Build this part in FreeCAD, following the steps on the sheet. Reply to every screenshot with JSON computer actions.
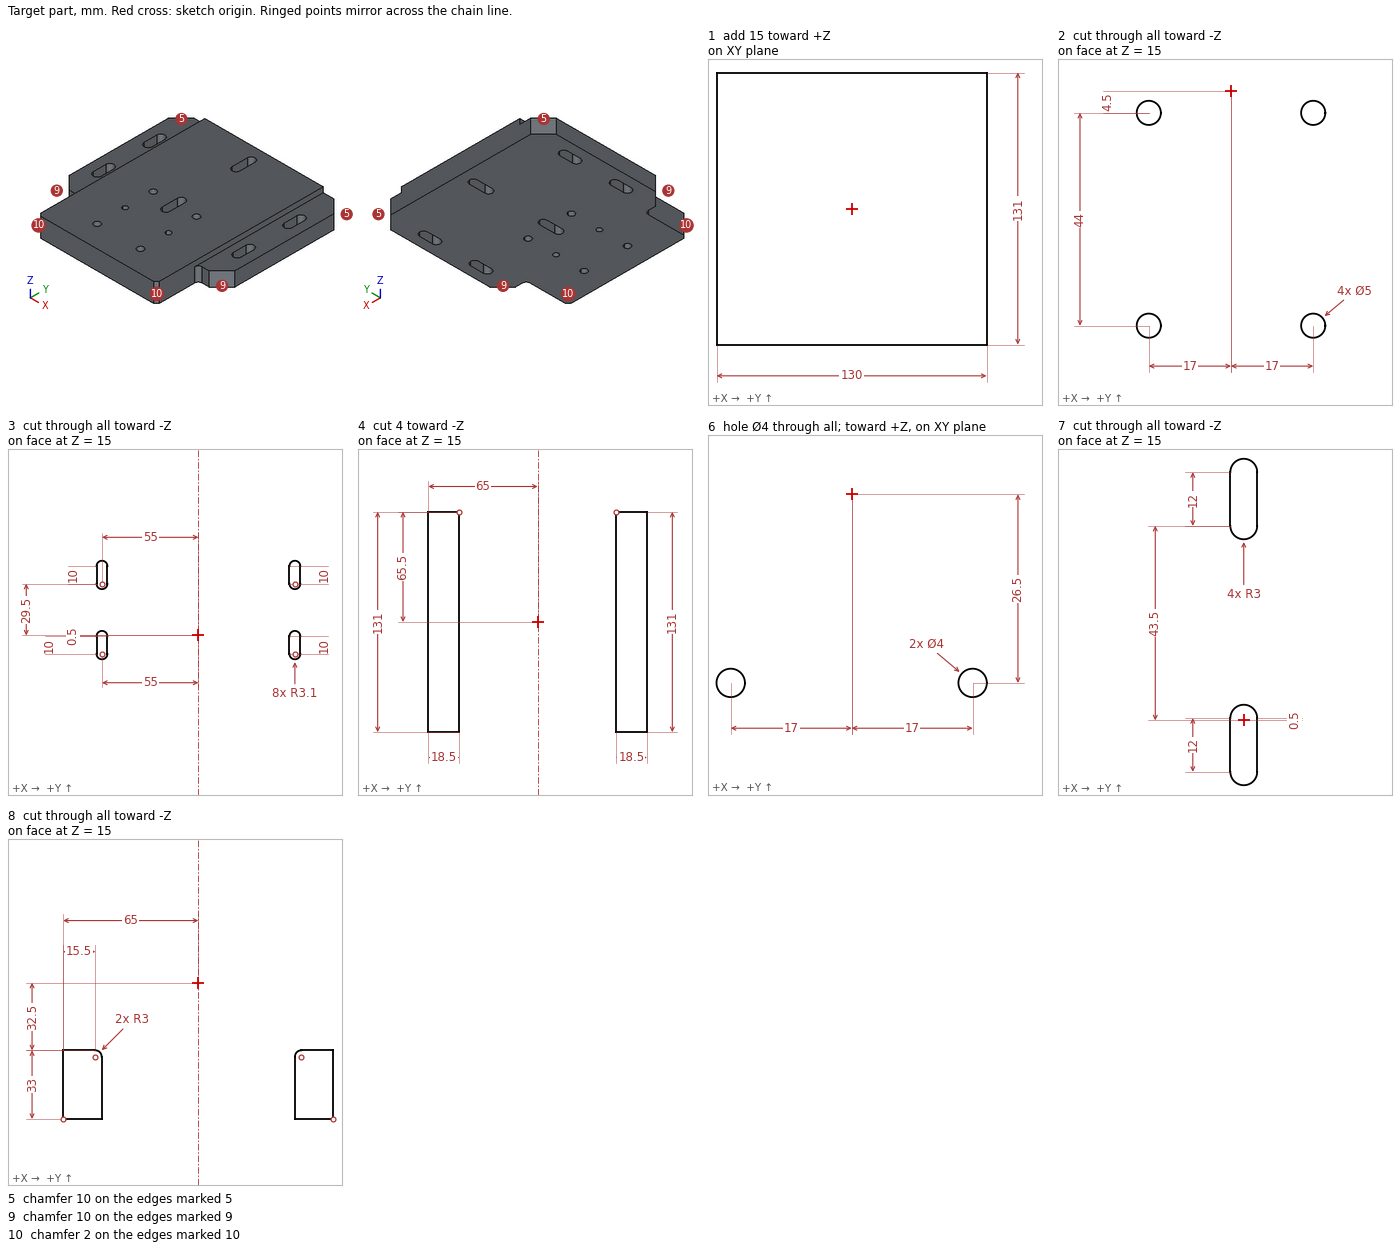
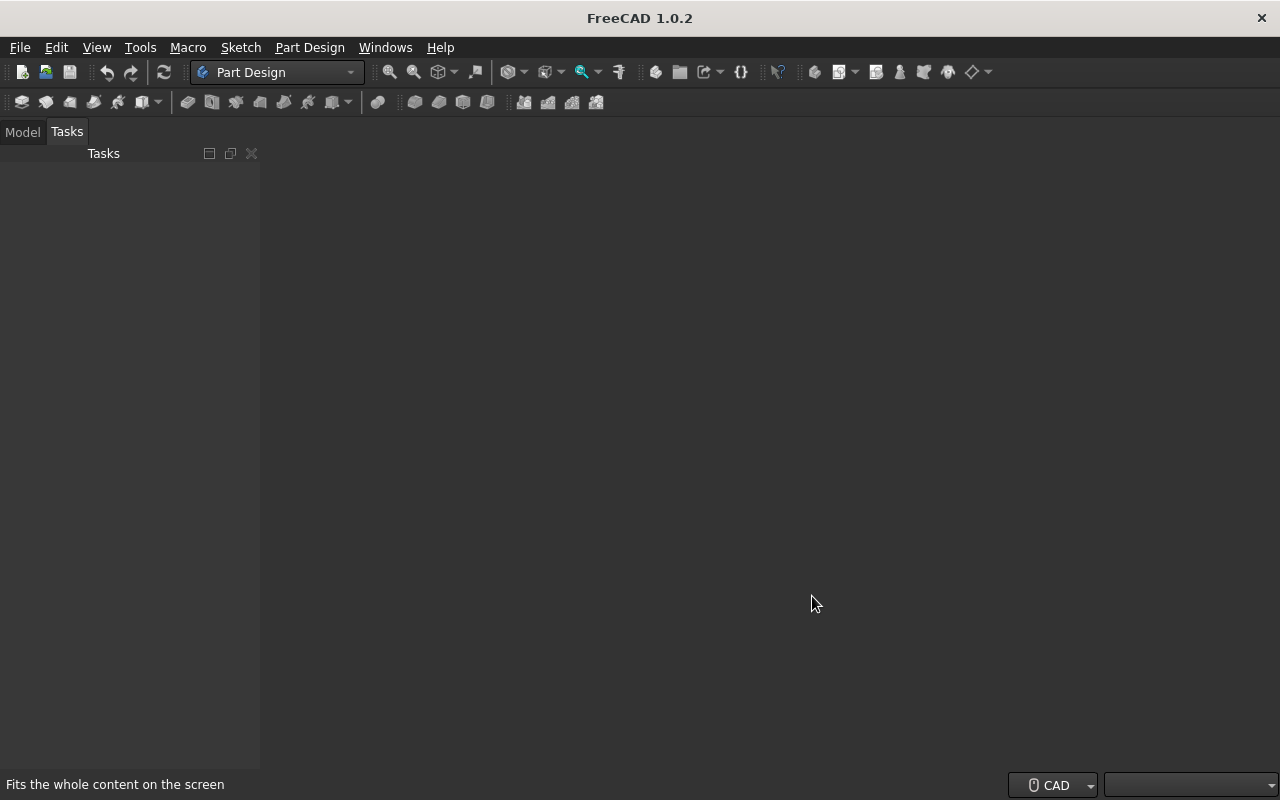
{"action": "key", "text": "ctrl+n"}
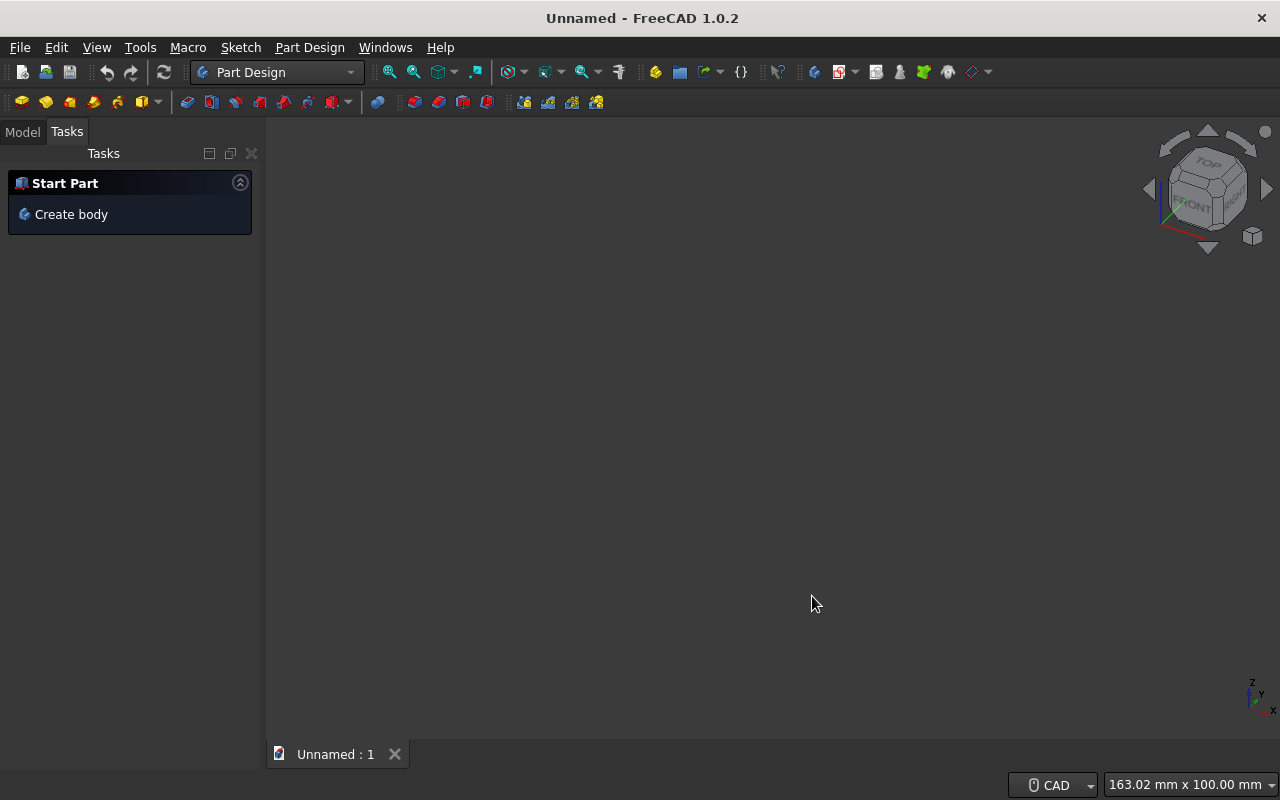
{"action": "left_click", "coordinate": [840, 72]}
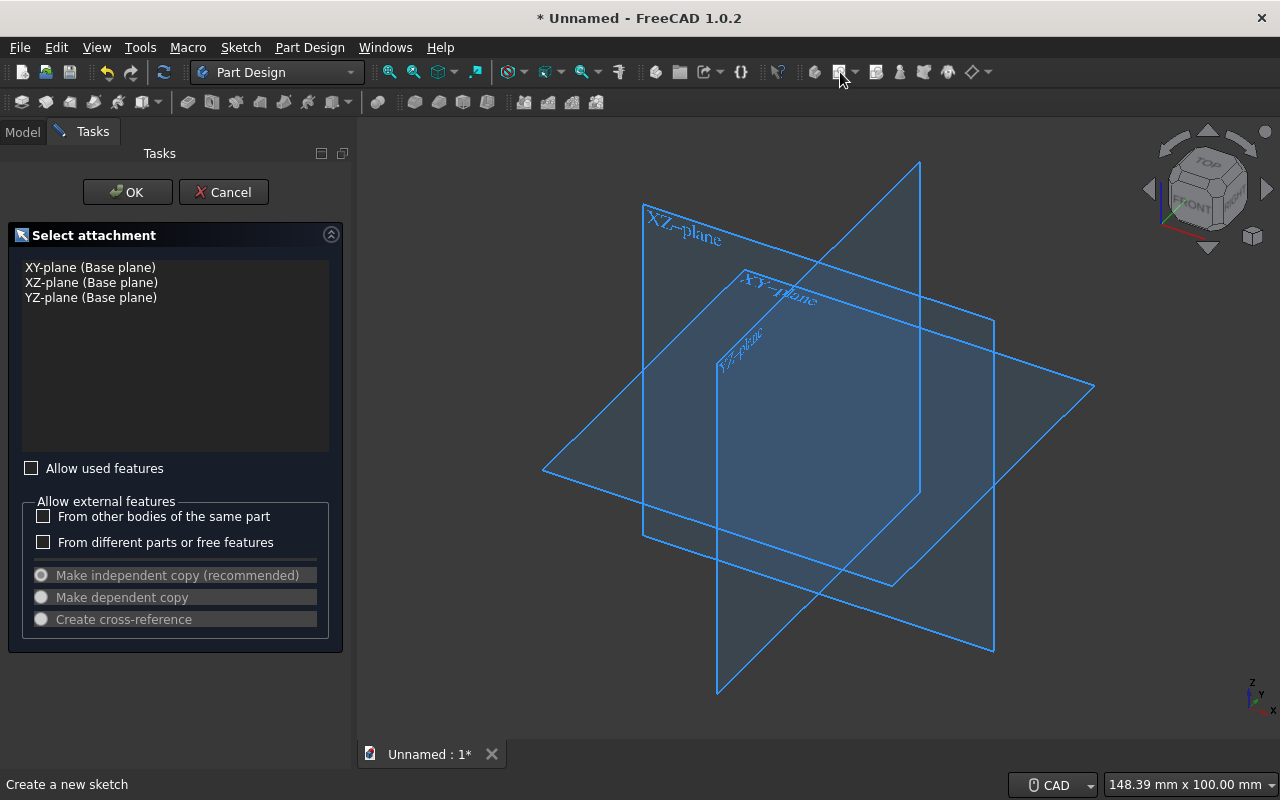
{"action": "left_click", "coordinate": [82, 268]}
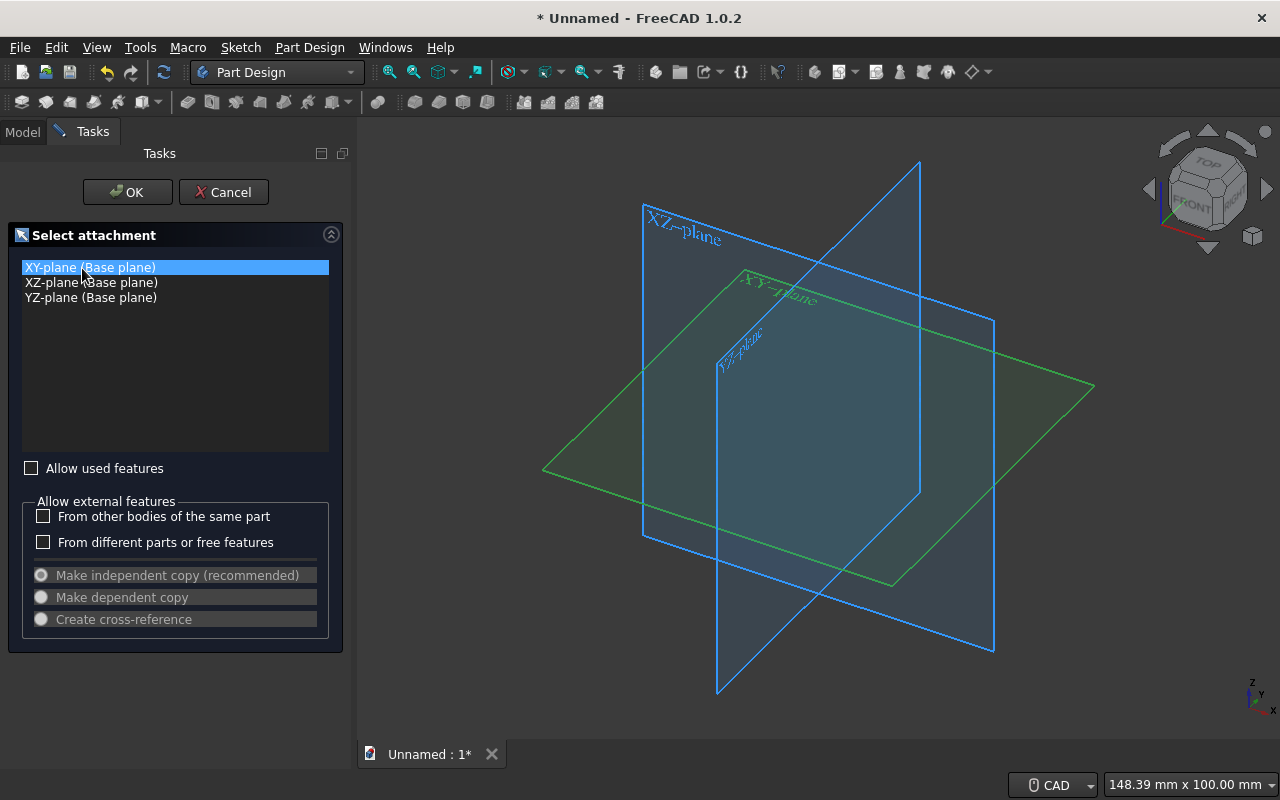
{"action": "left_click", "coordinate": [128, 192]}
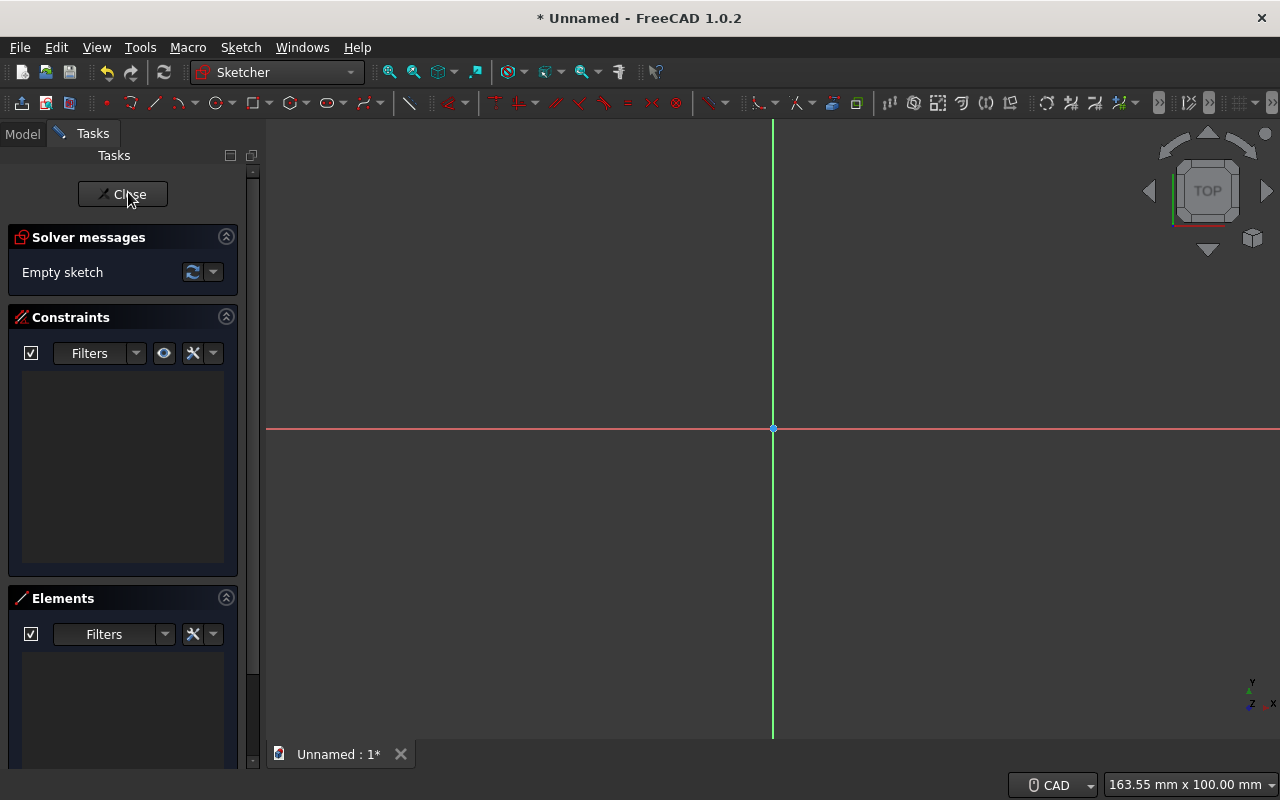
{"action": "scroll", "coordinate": [649, 429], "scroll_direction": "down", "scroll_amount": 4}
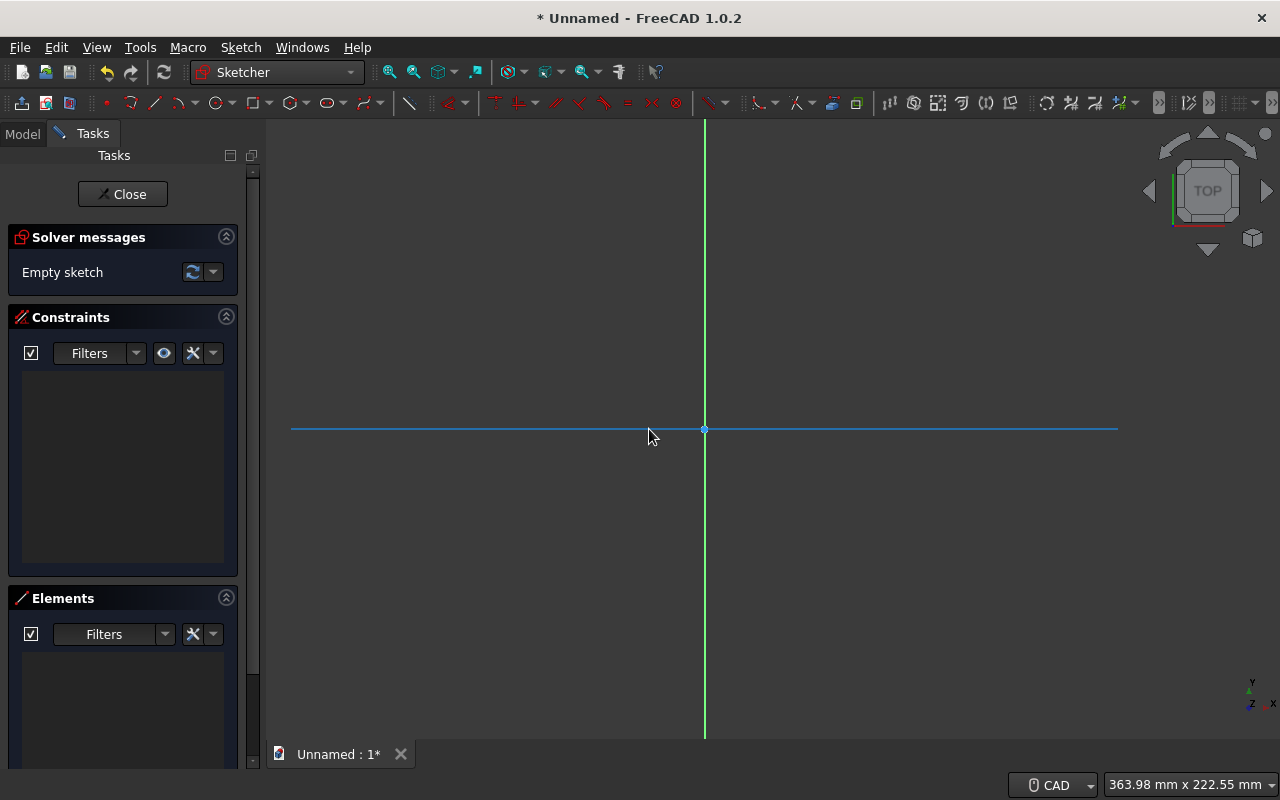
{"action": "left_click", "coordinate": [272, 104]}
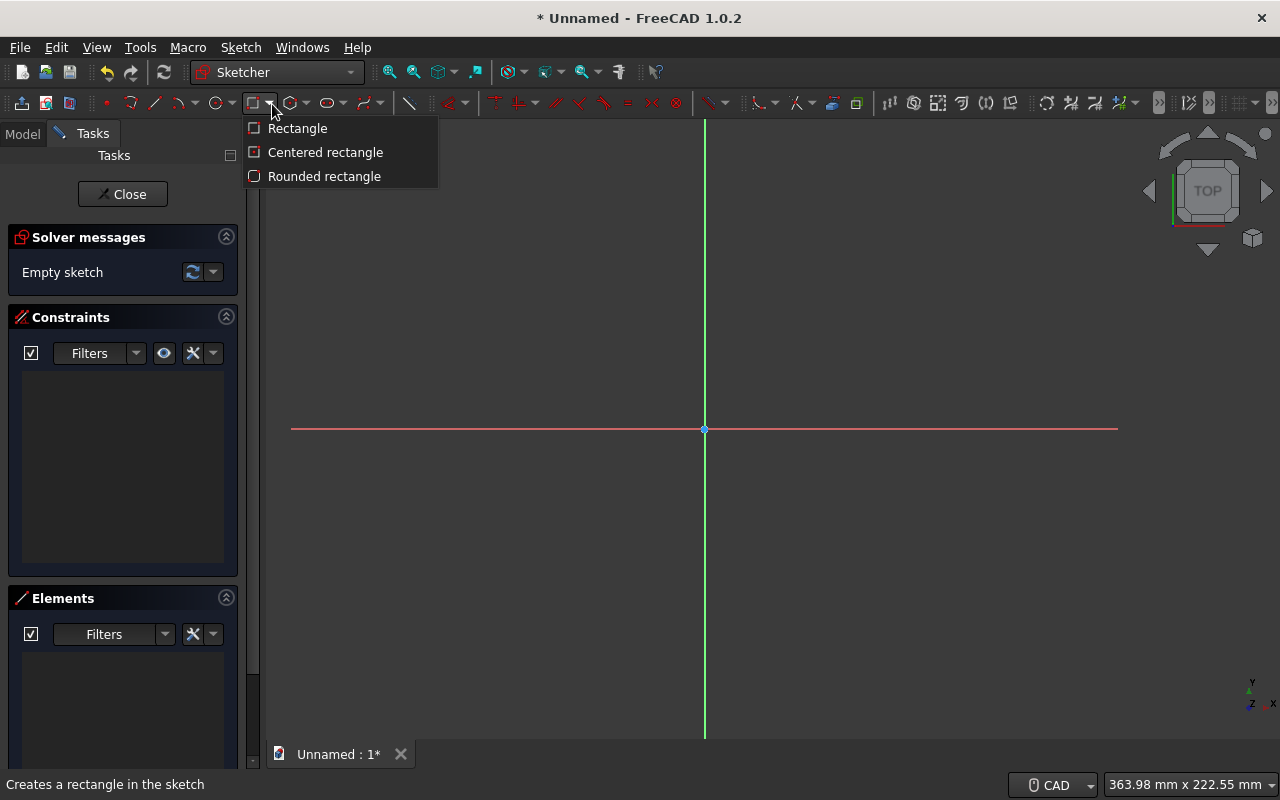
{"action": "left_click", "coordinate": [340, 152]}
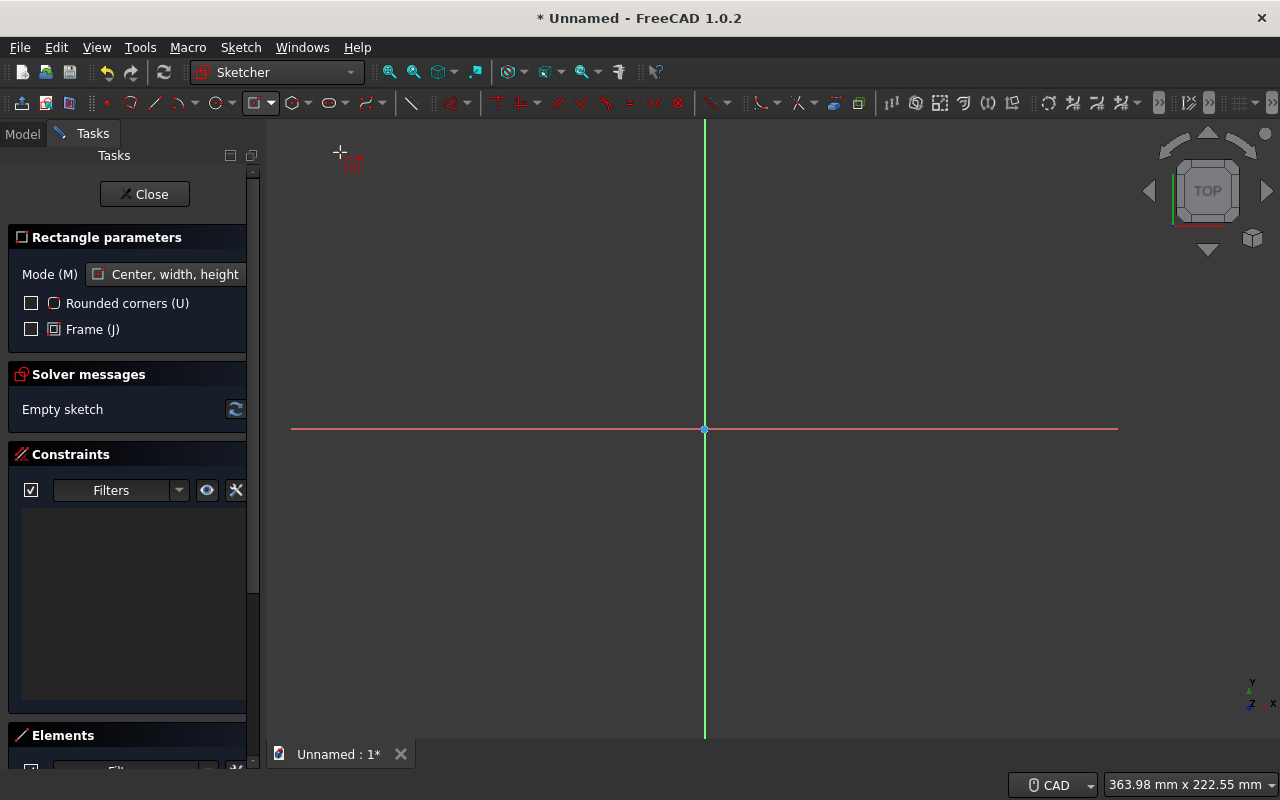
{"action": "left_click", "coordinate": [705, 429]}
{"action": "mouse_move", "coordinate": [886, 247]}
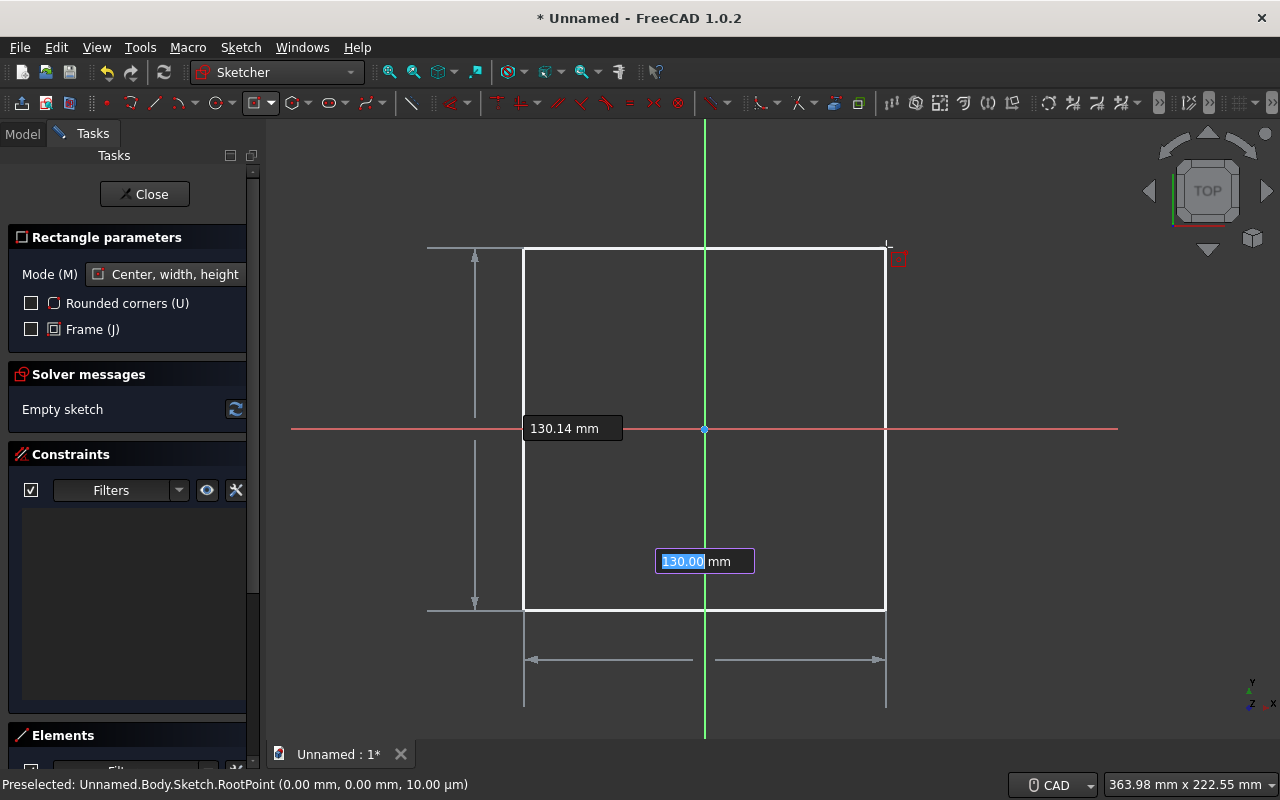
{"action": "type", "text": "130"}
{"action": "key", "text": "Tab"}
{"action": "type", "text": "131"}
{"action": "key", "text": "Return"}
{"action": "key", "text": "Escape"}